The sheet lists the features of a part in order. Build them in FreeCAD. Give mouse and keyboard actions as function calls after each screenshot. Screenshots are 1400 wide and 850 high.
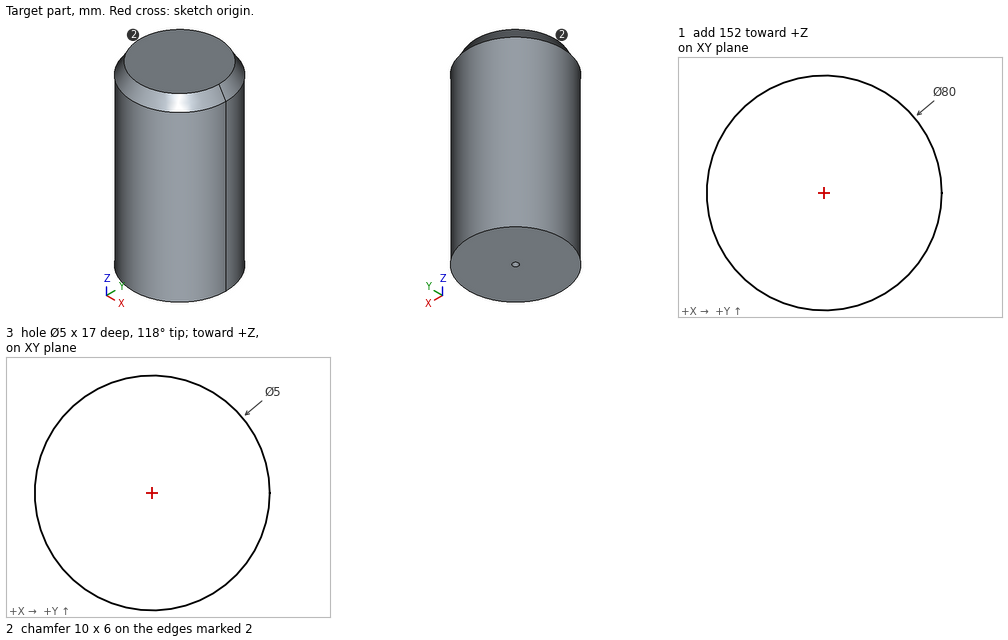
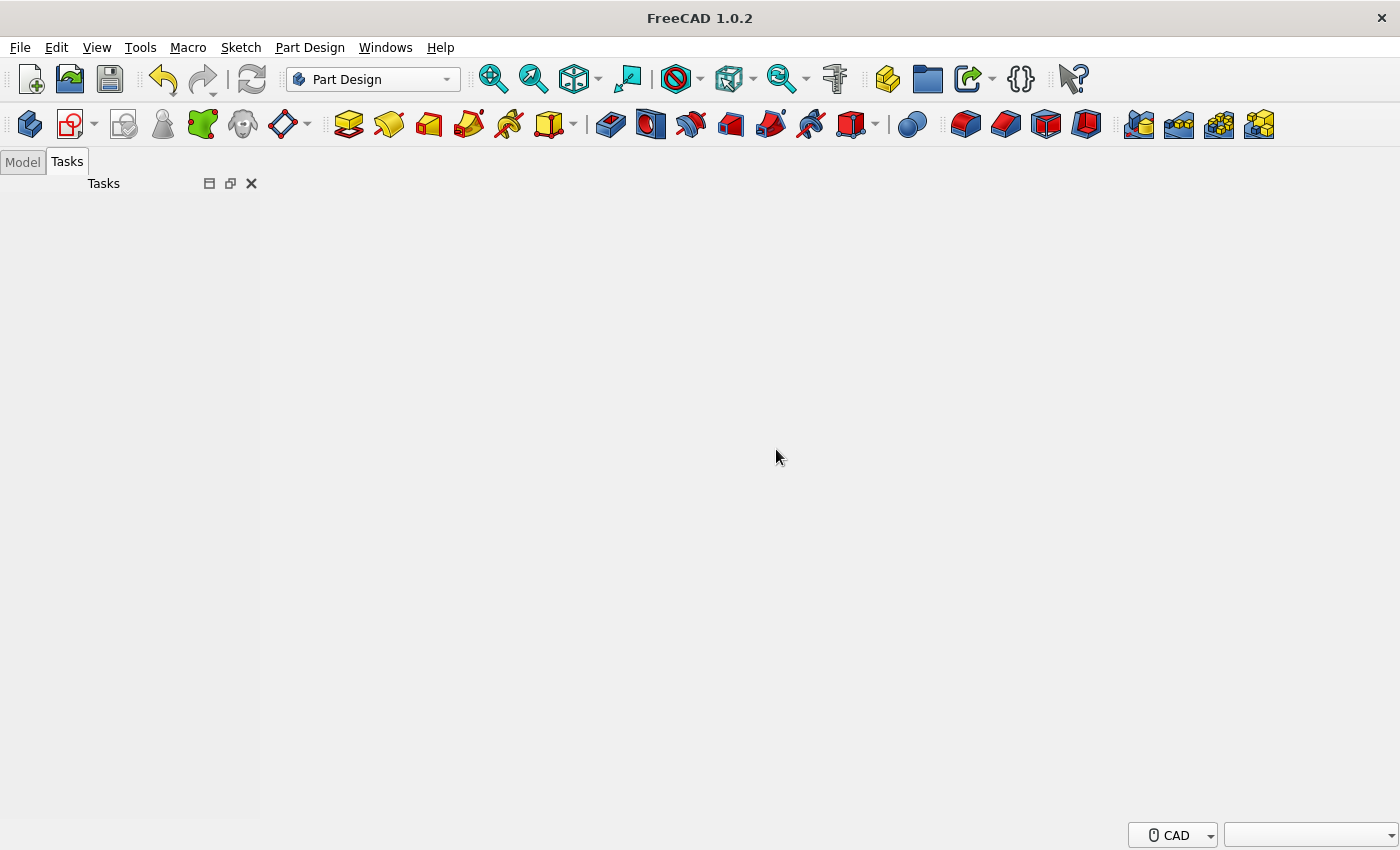
click(30, 80)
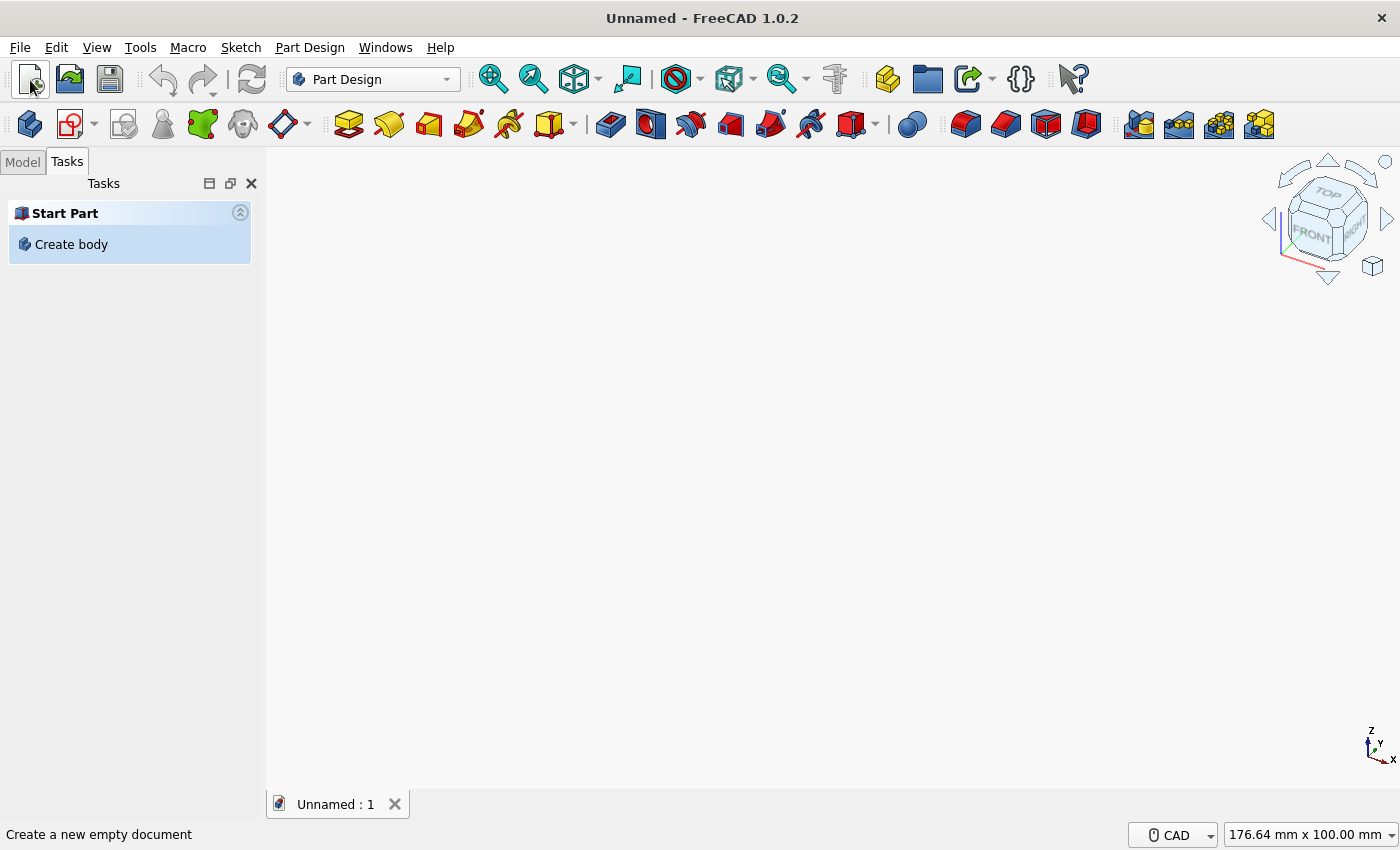
click(70, 124)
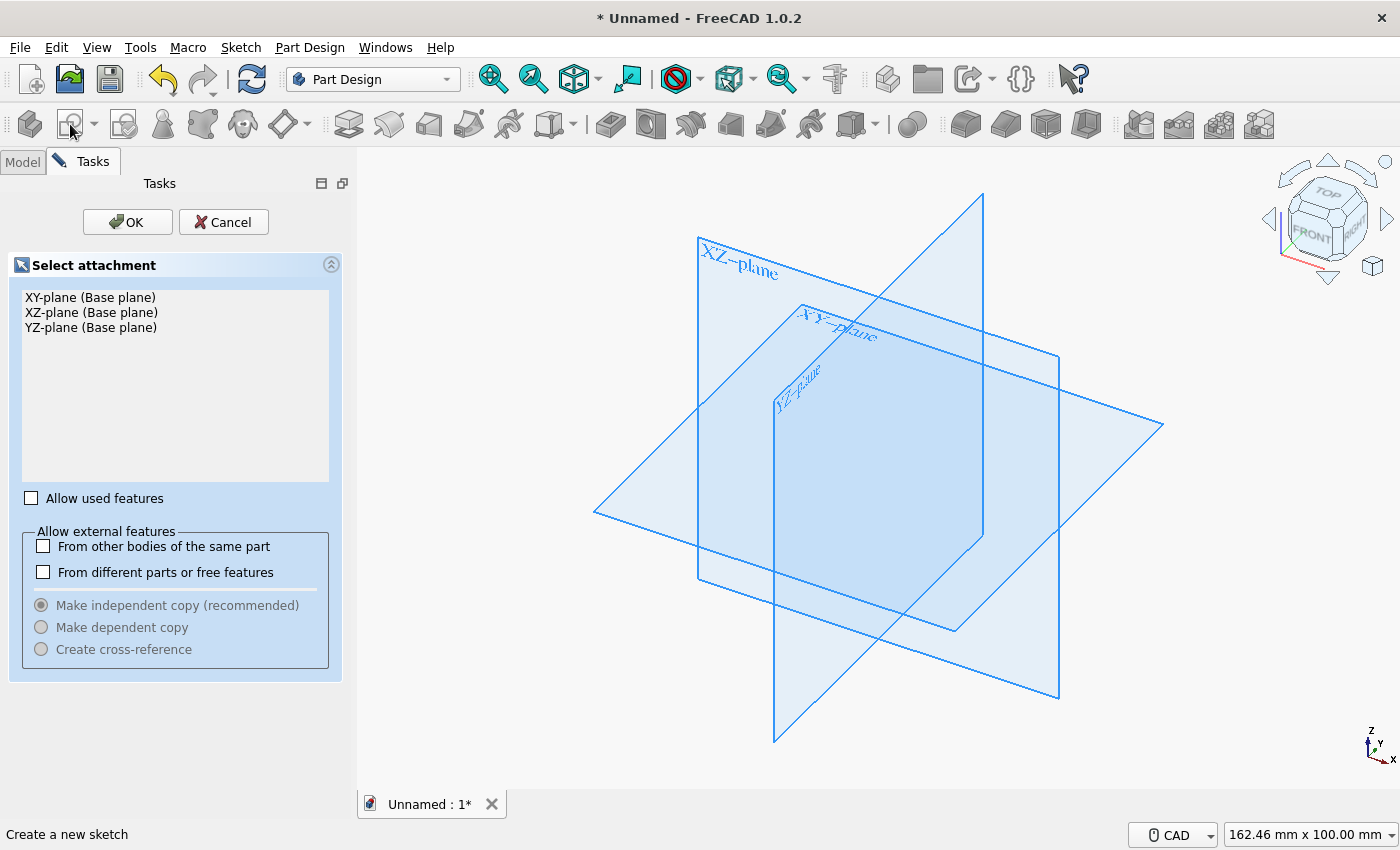
click(82, 298)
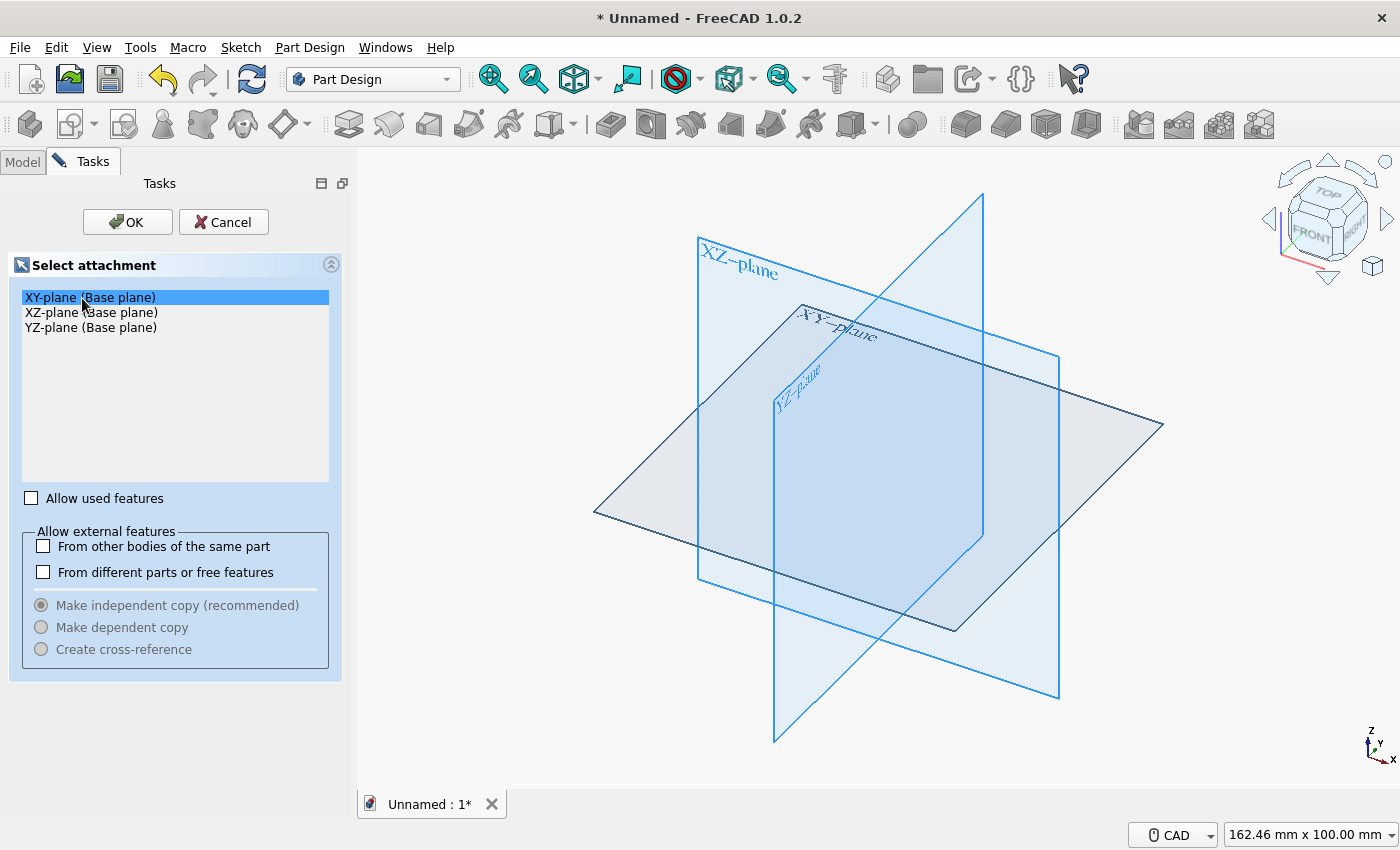
click(128, 222)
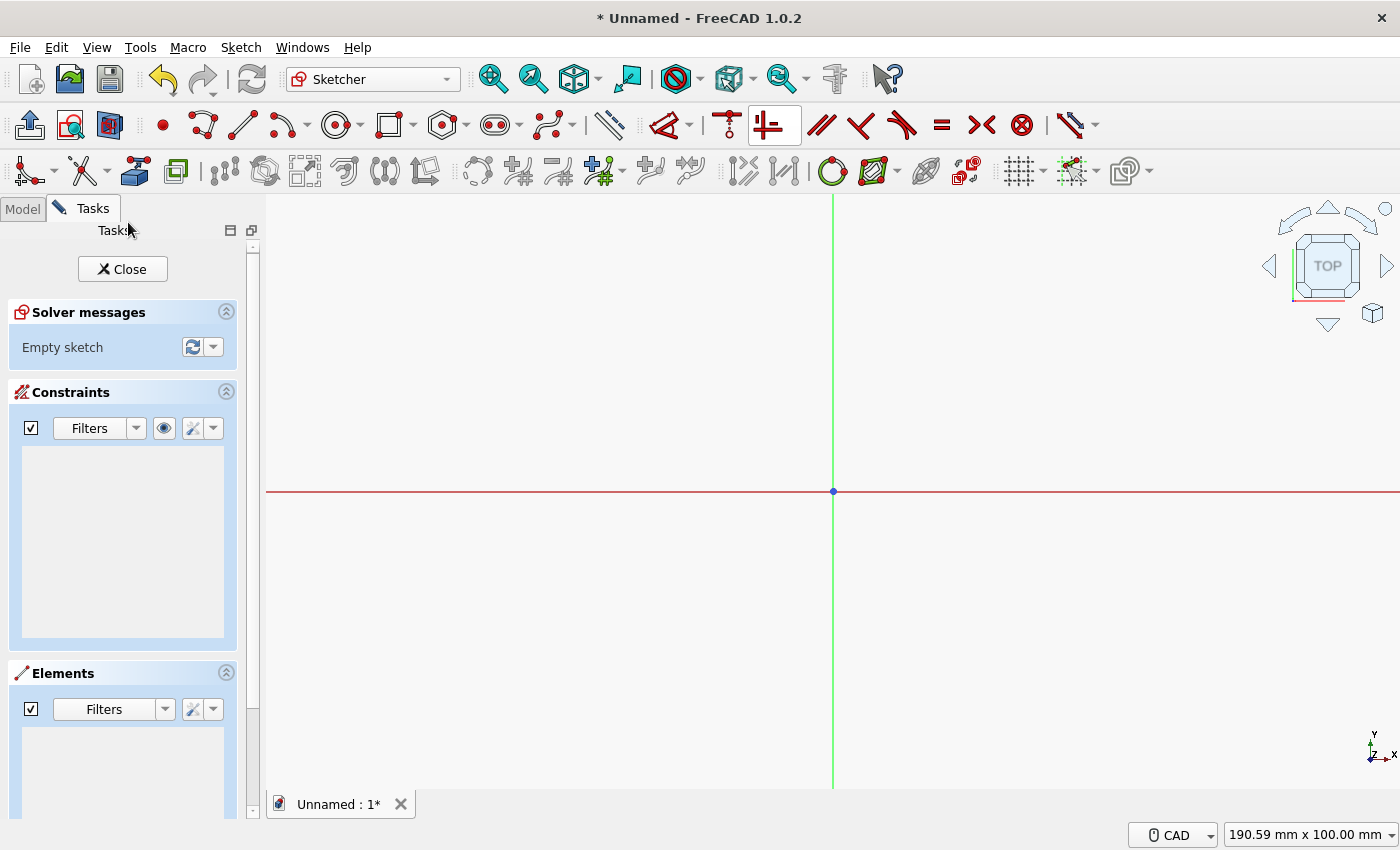
click(336, 126)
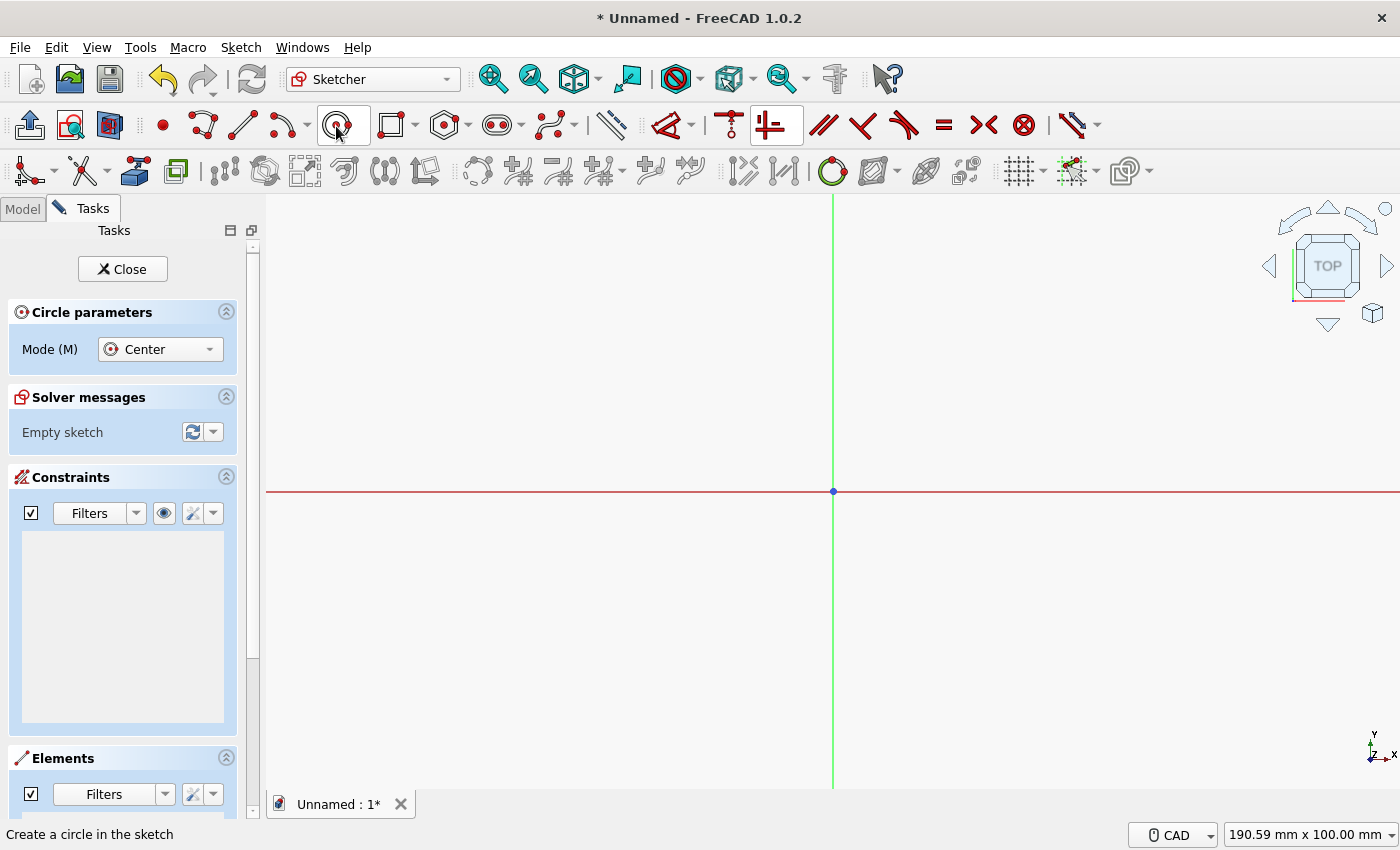
click(833, 492)
click(1001, 323)
key(Escape)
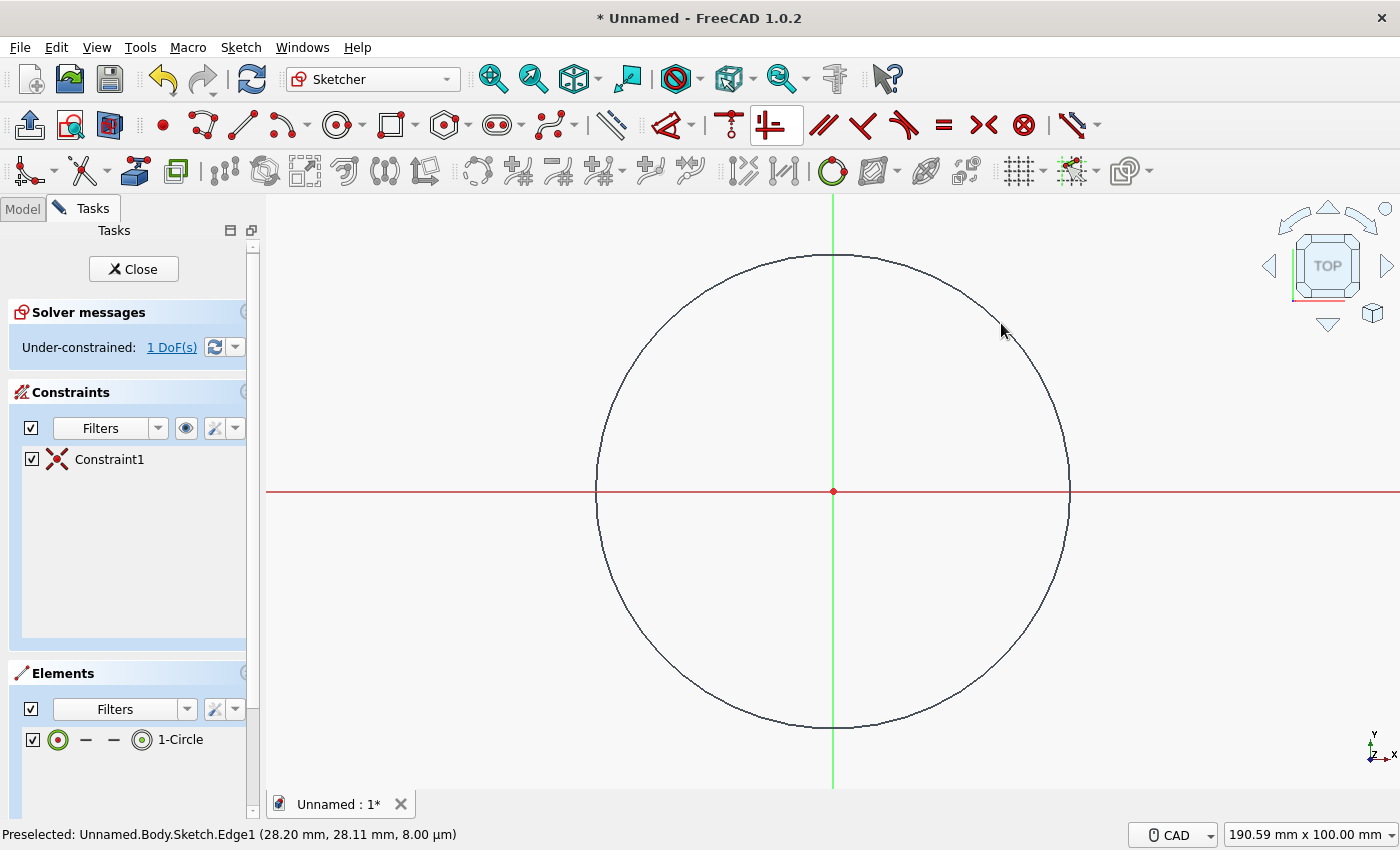
click(666, 126)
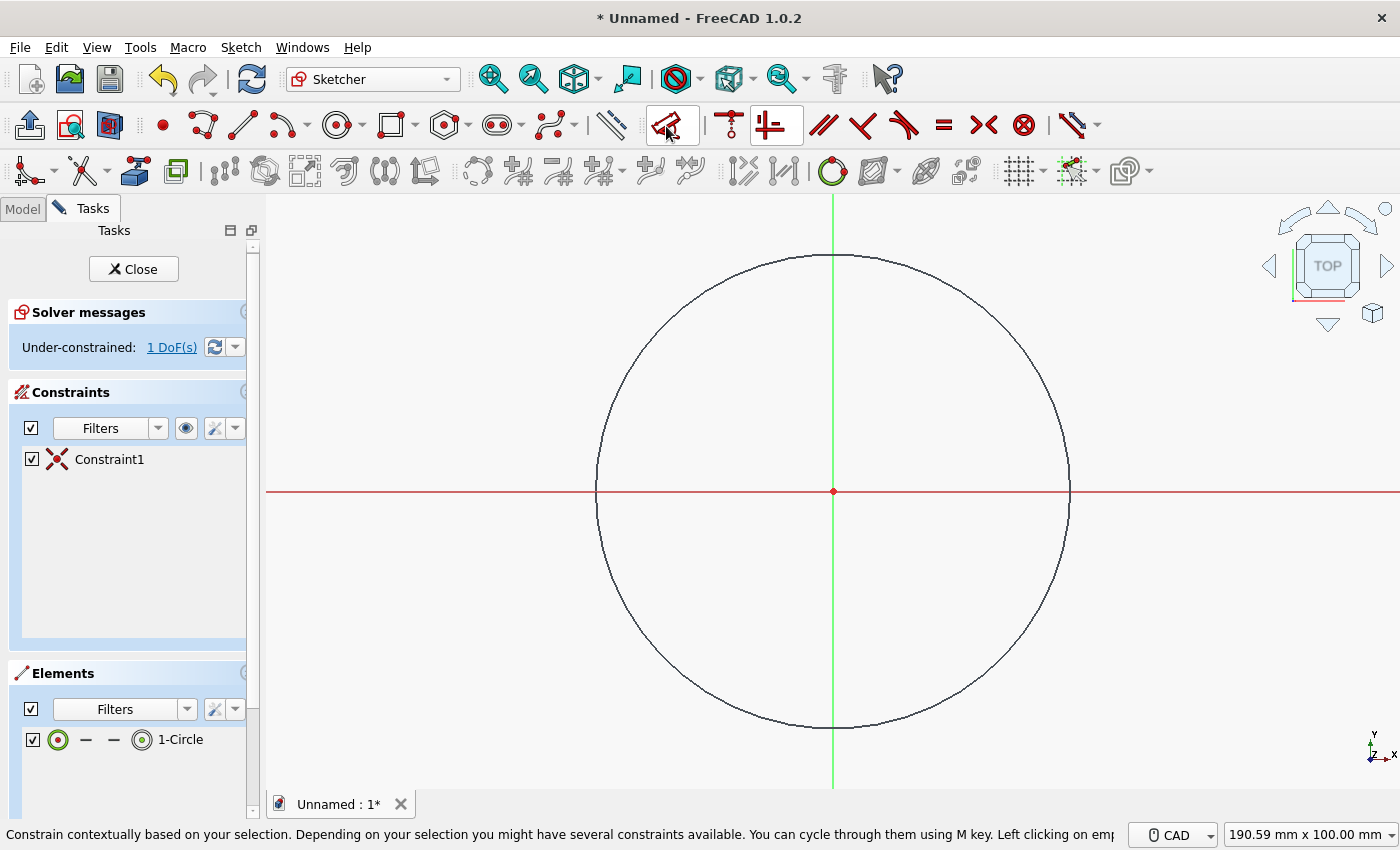
click(1000, 323)
click(1023, 300)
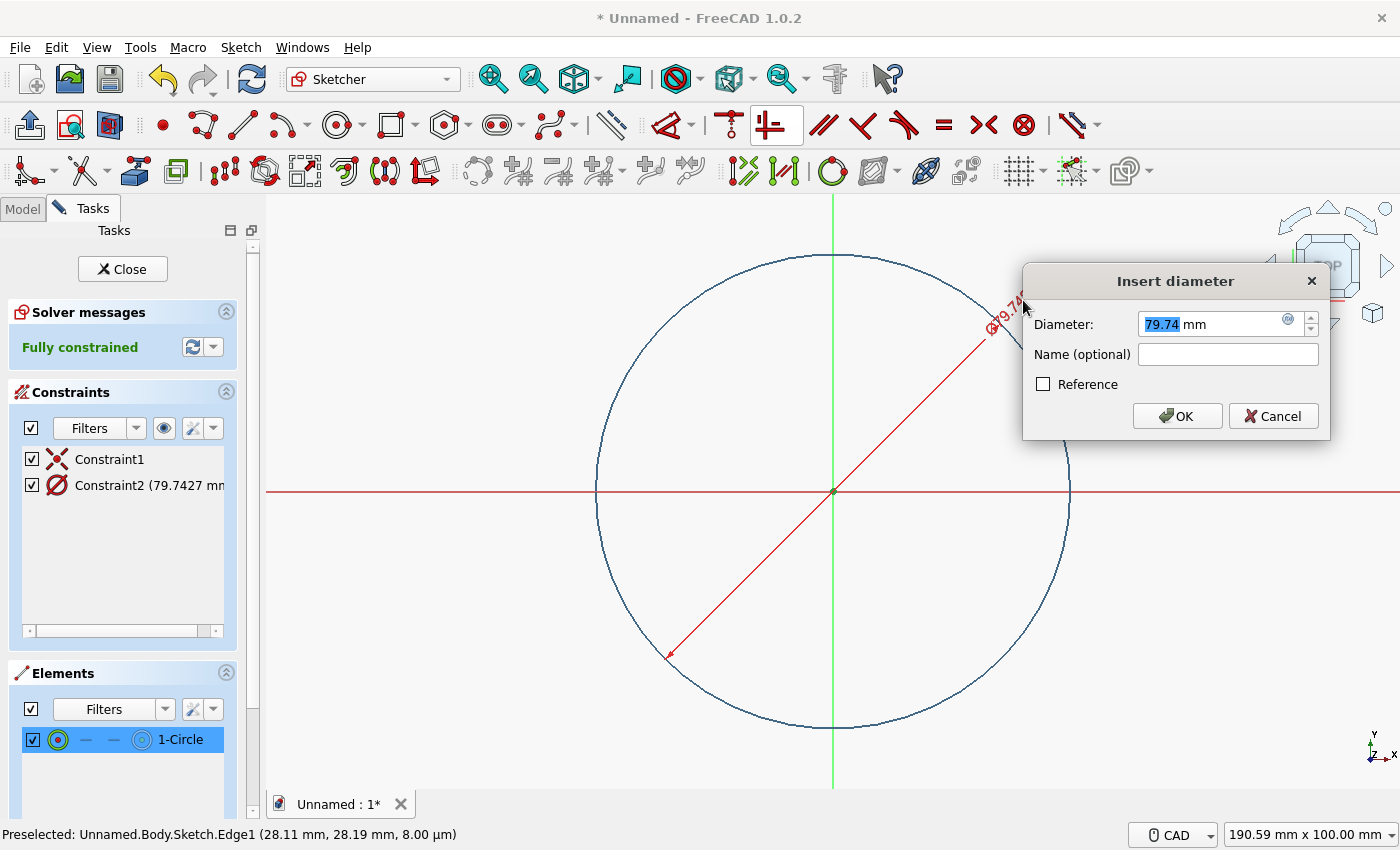
text(80)
key(Return)
key(Escape)